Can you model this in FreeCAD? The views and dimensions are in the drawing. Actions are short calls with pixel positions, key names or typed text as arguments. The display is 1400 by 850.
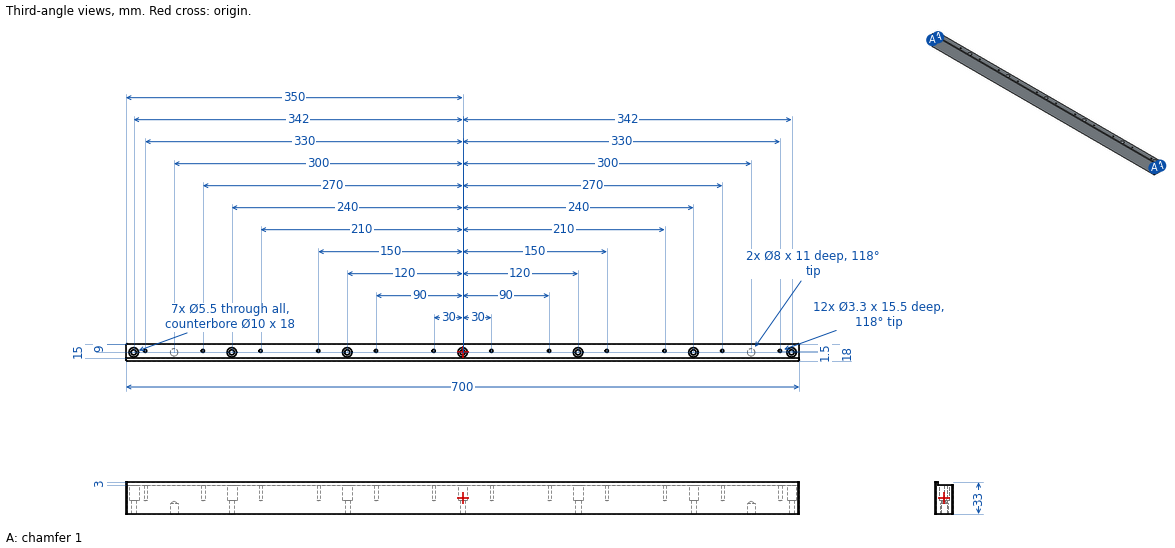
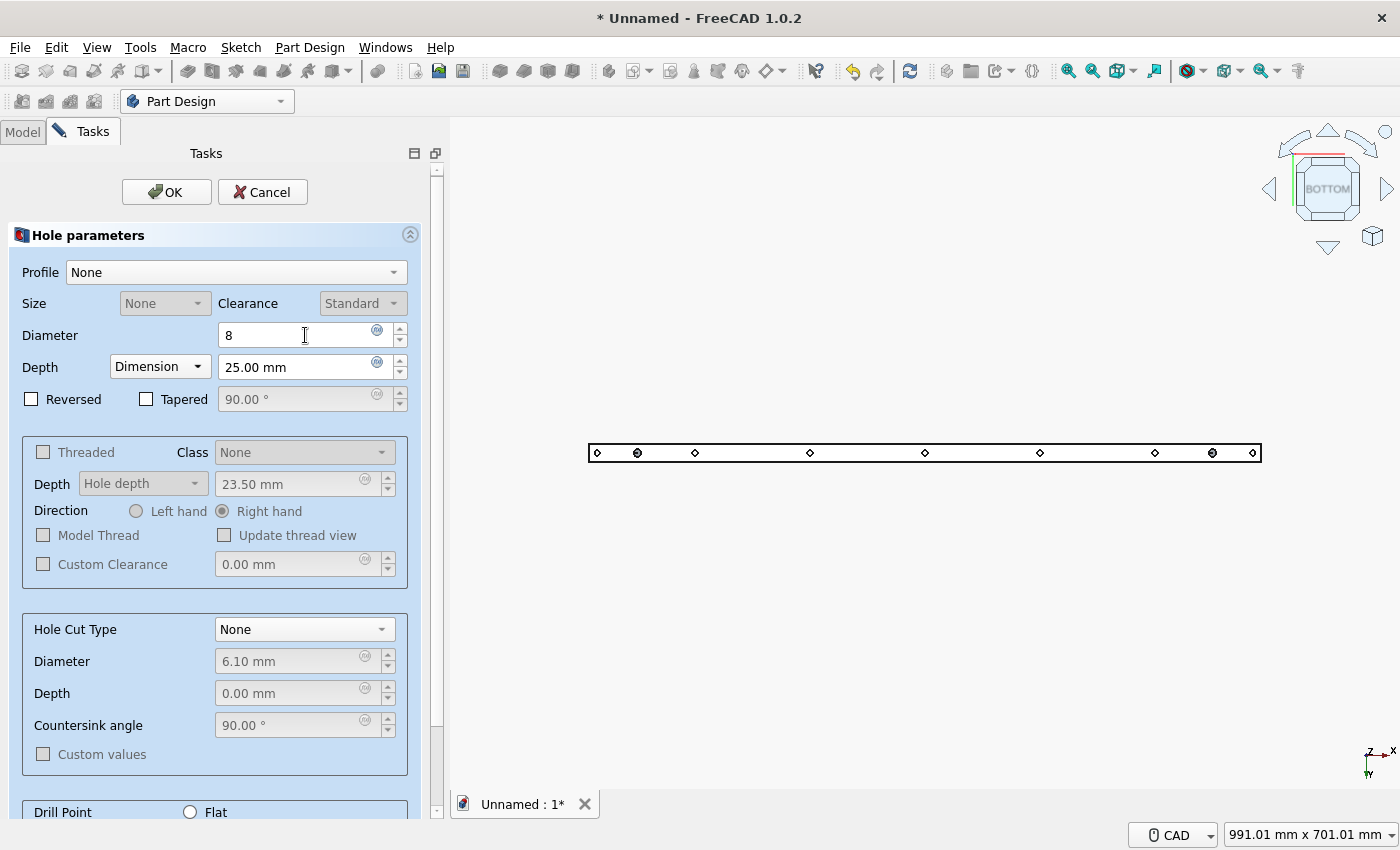
triple_click(305, 367)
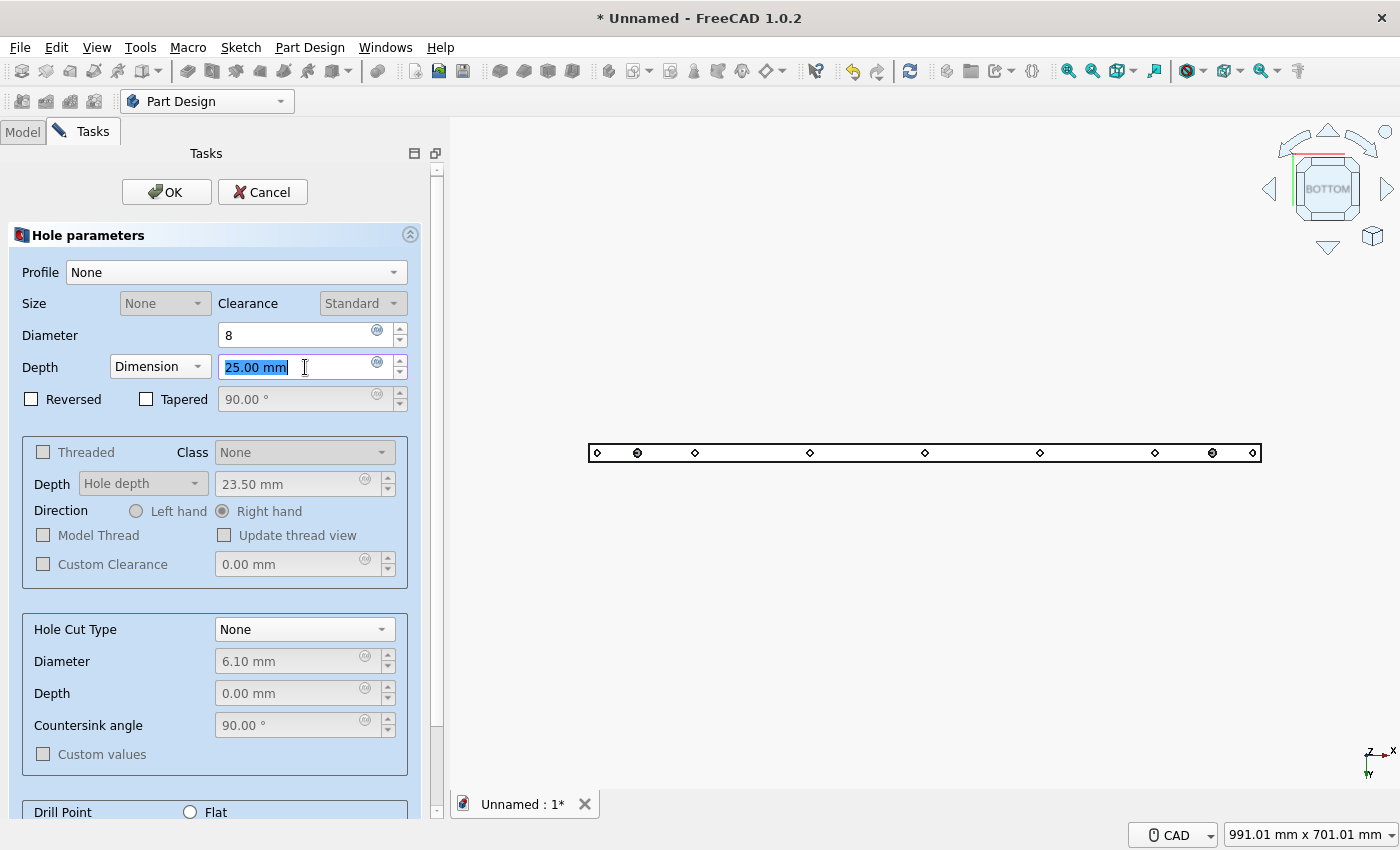
text(11)
key(Tab)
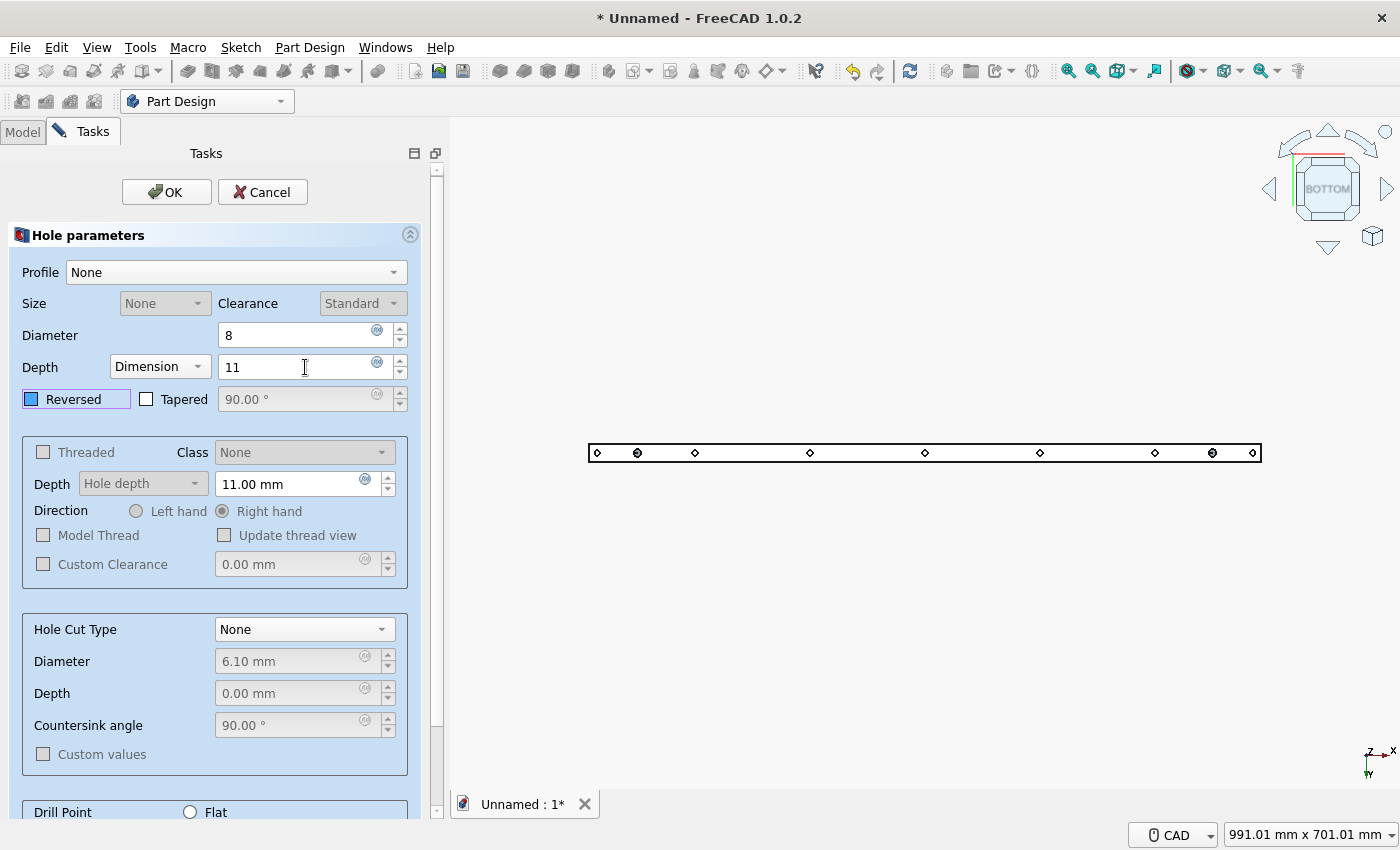
click(167, 192)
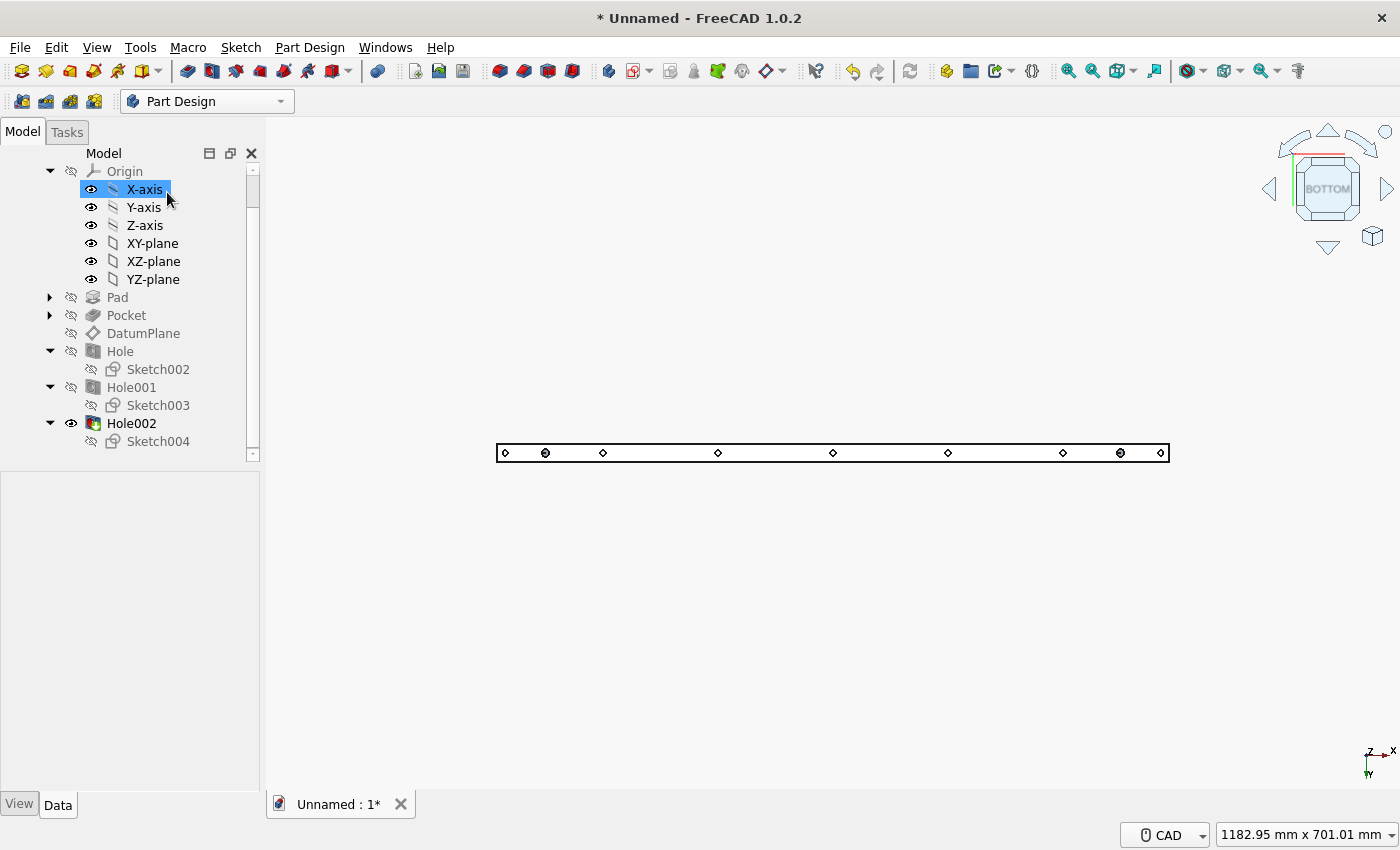
key(0)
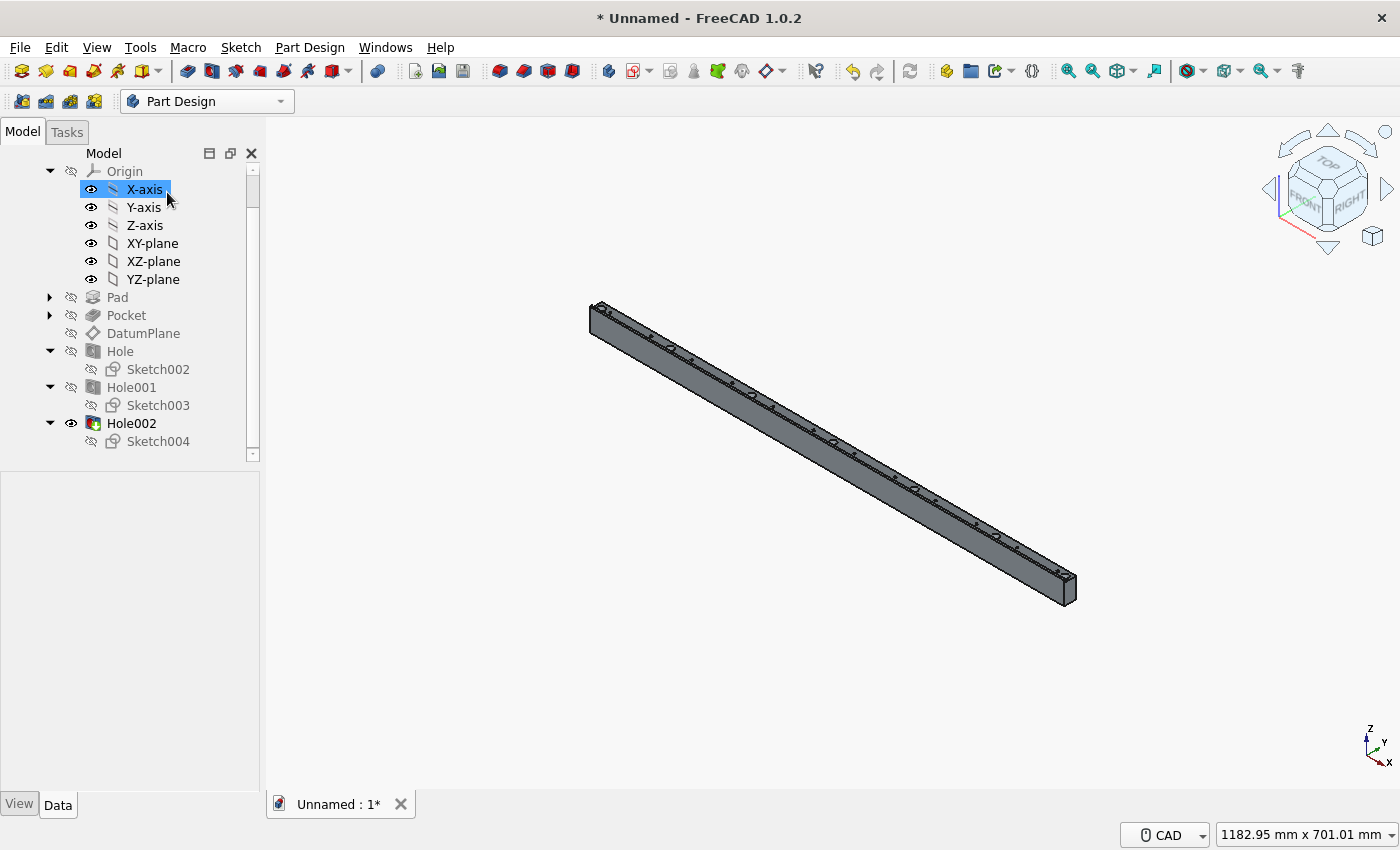
click(1064, 592)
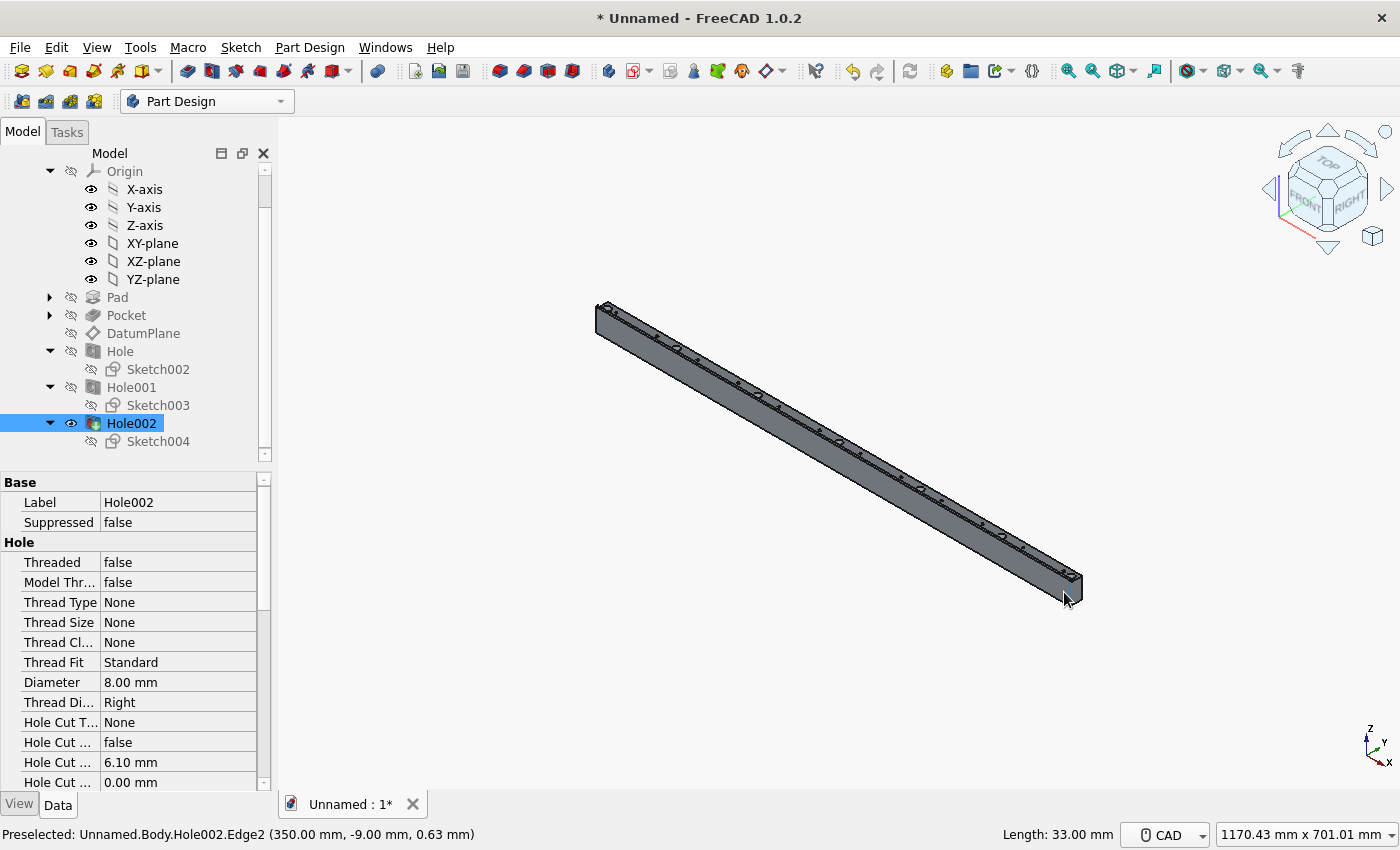
key(2)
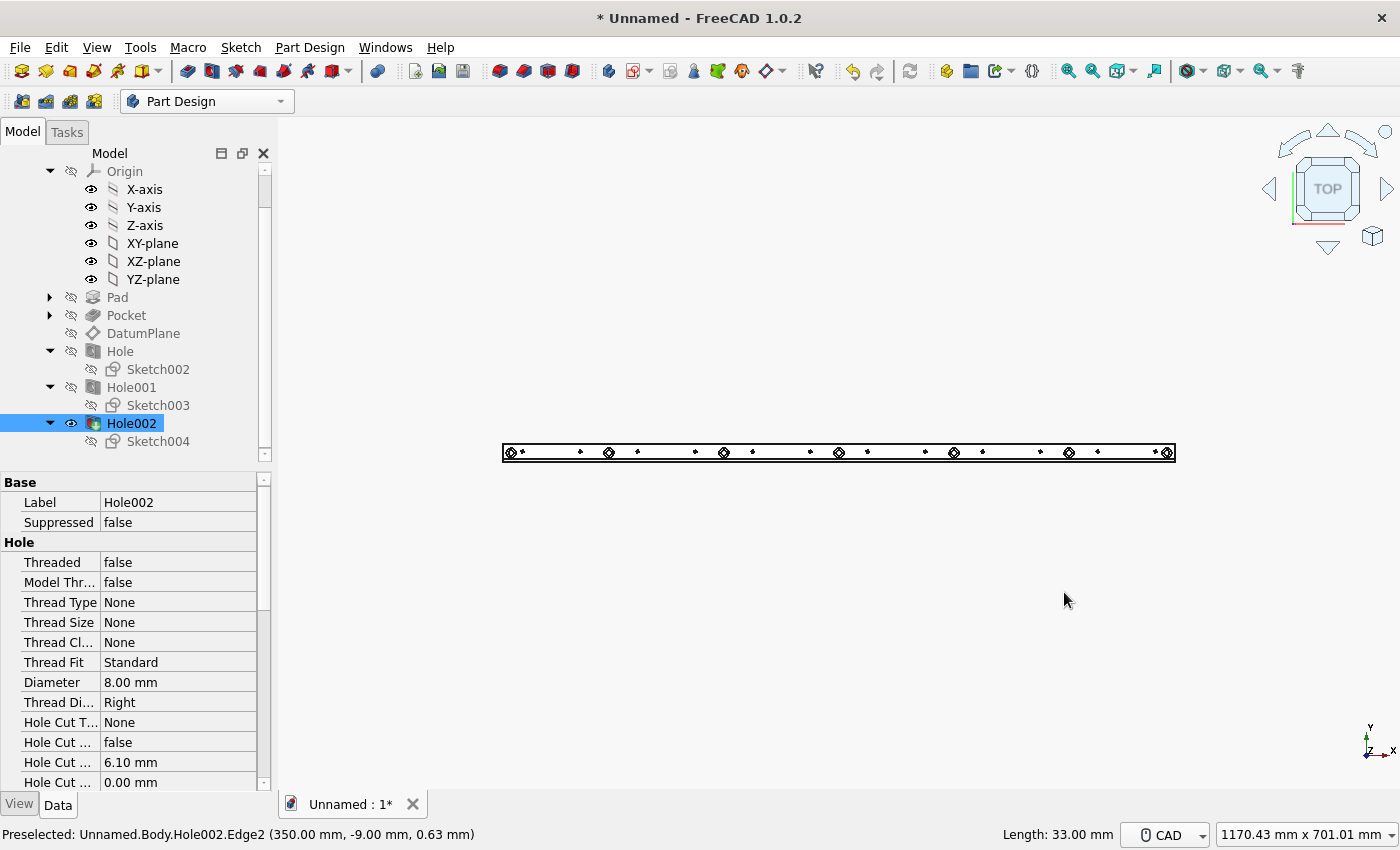
key(1)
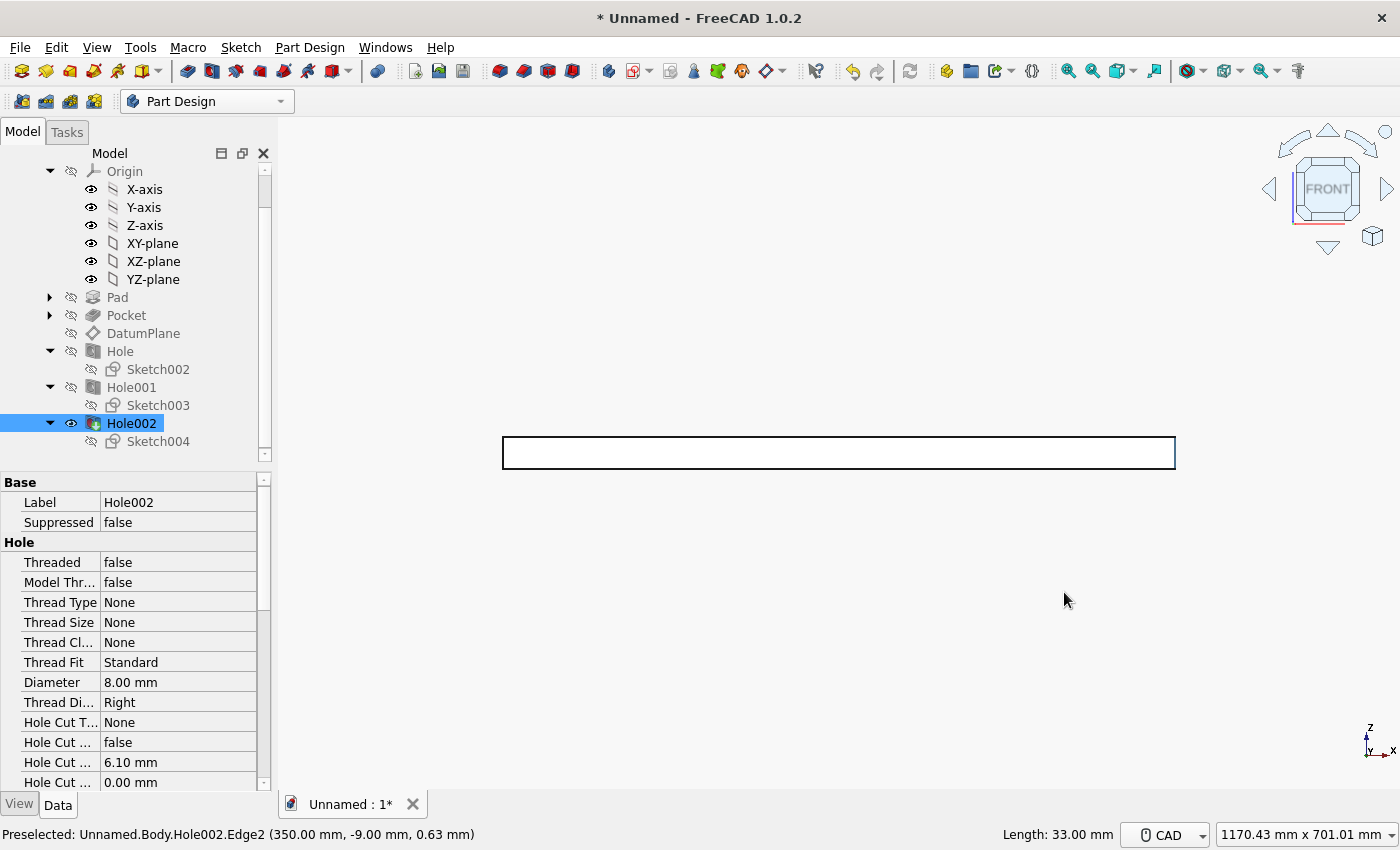
click(503, 452, ctrl)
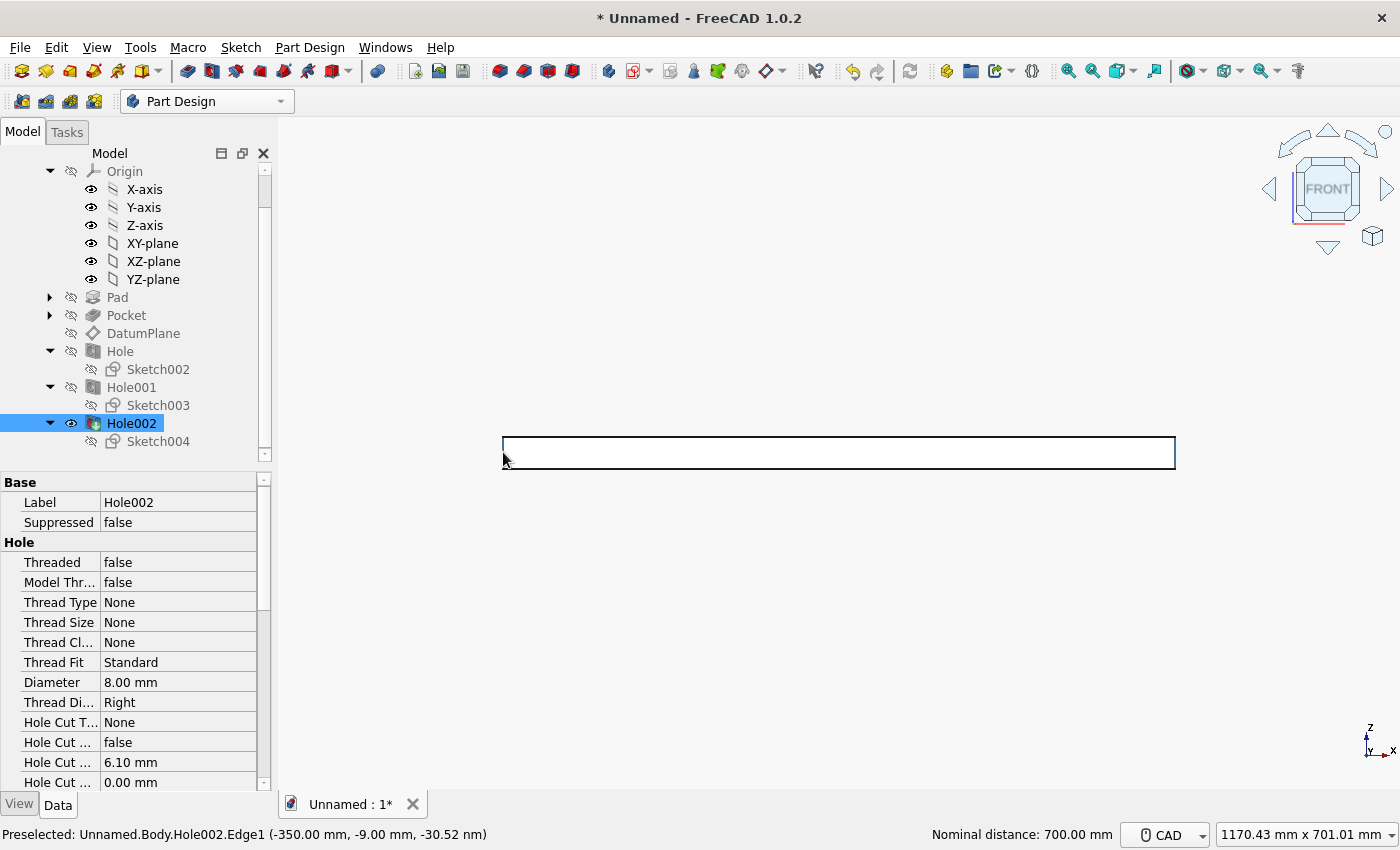
key(3)